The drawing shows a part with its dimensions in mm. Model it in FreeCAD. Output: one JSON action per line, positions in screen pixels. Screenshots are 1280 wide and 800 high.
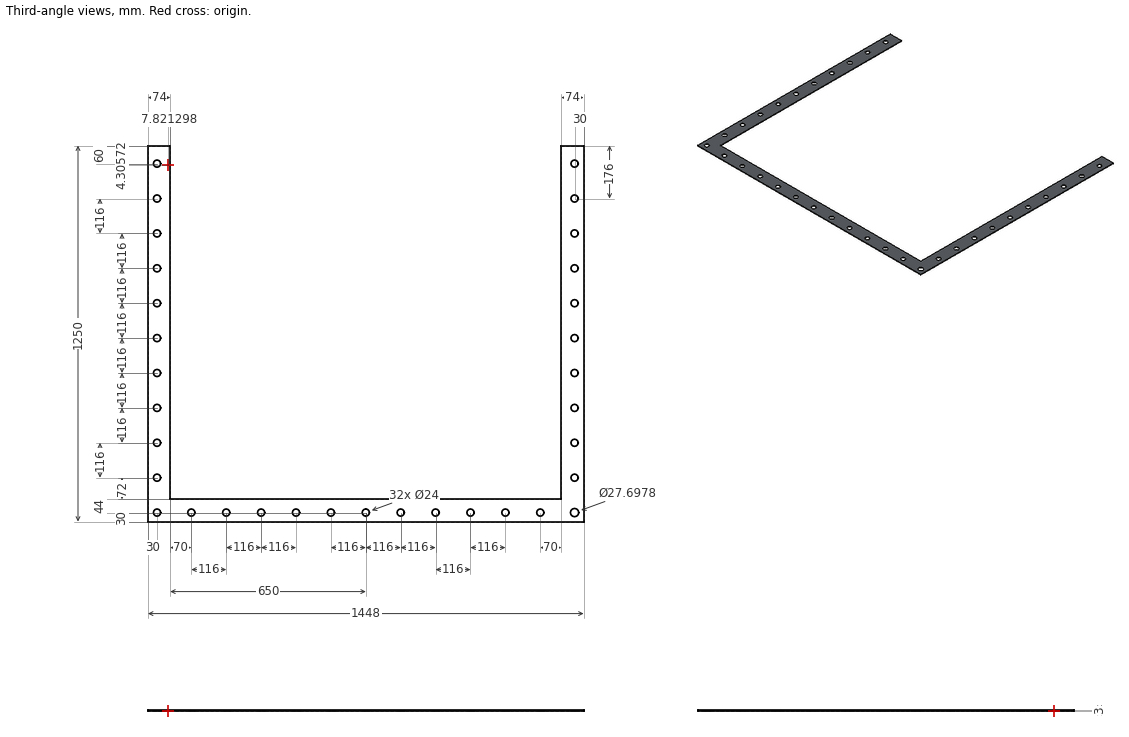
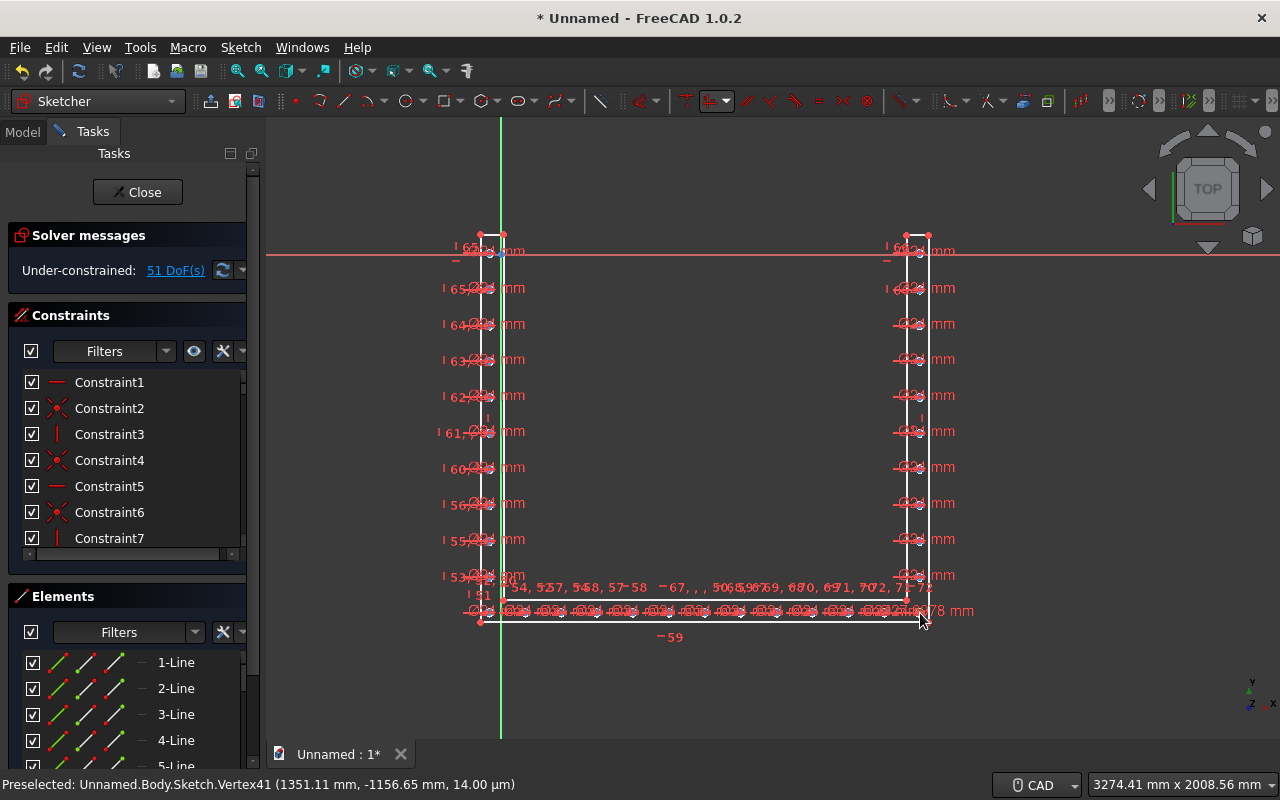
{"action": "left_click", "coordinate": [920, 577]}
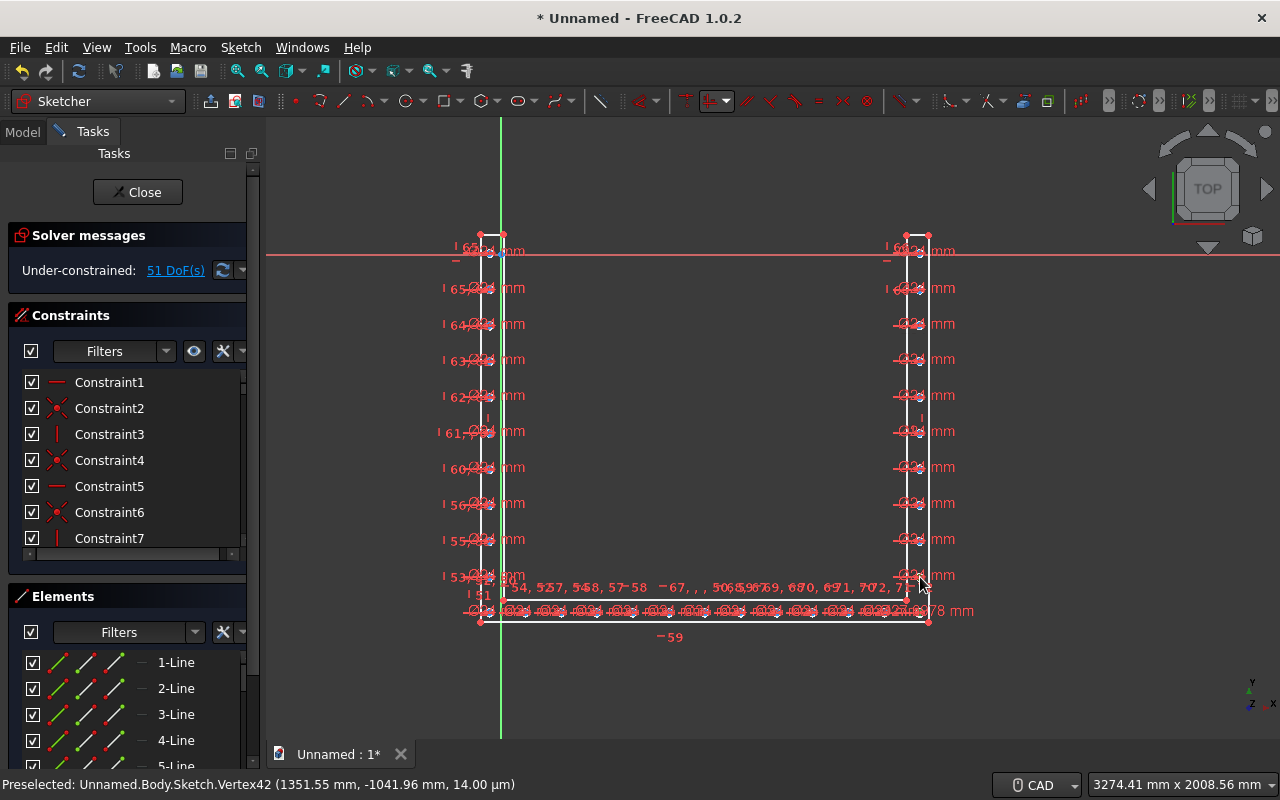
{"action": "left_click", "coordinate": [728, 102]}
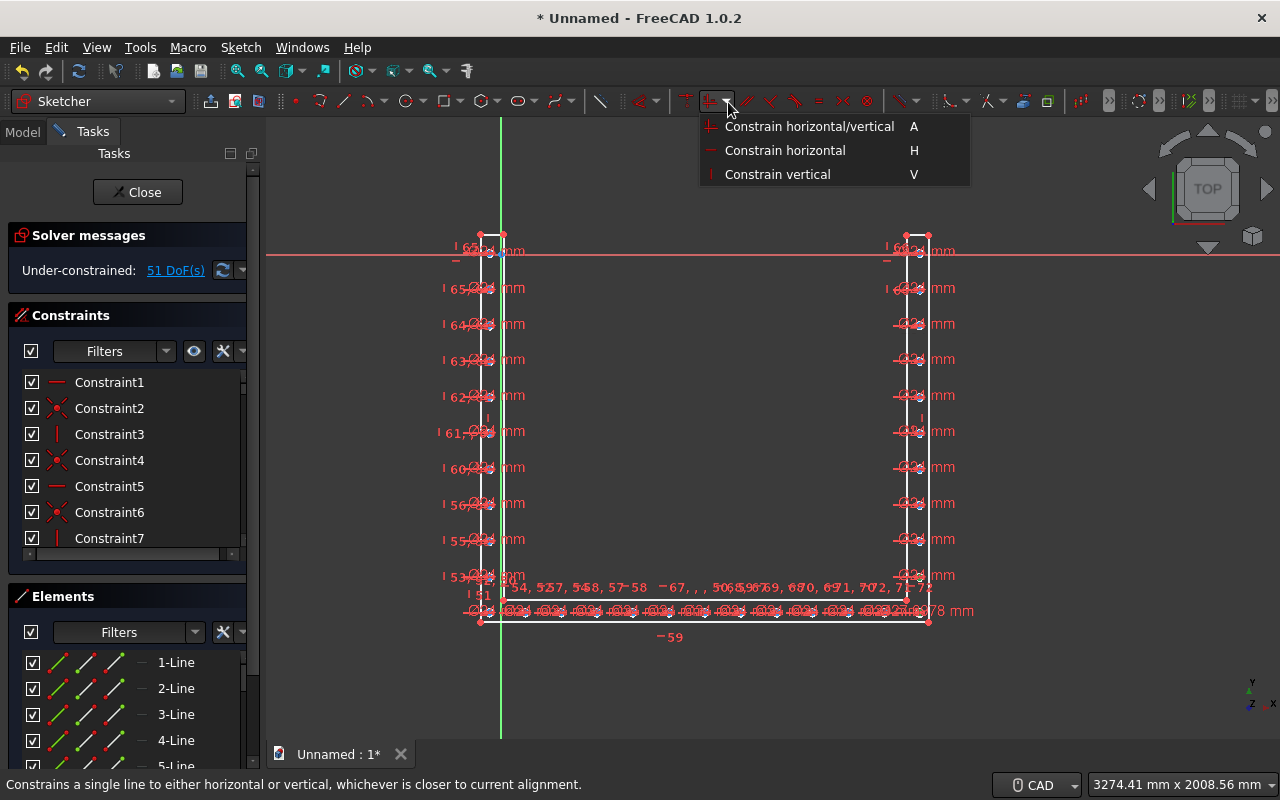
{"action": "left_click", "coordinate": [835, 174]}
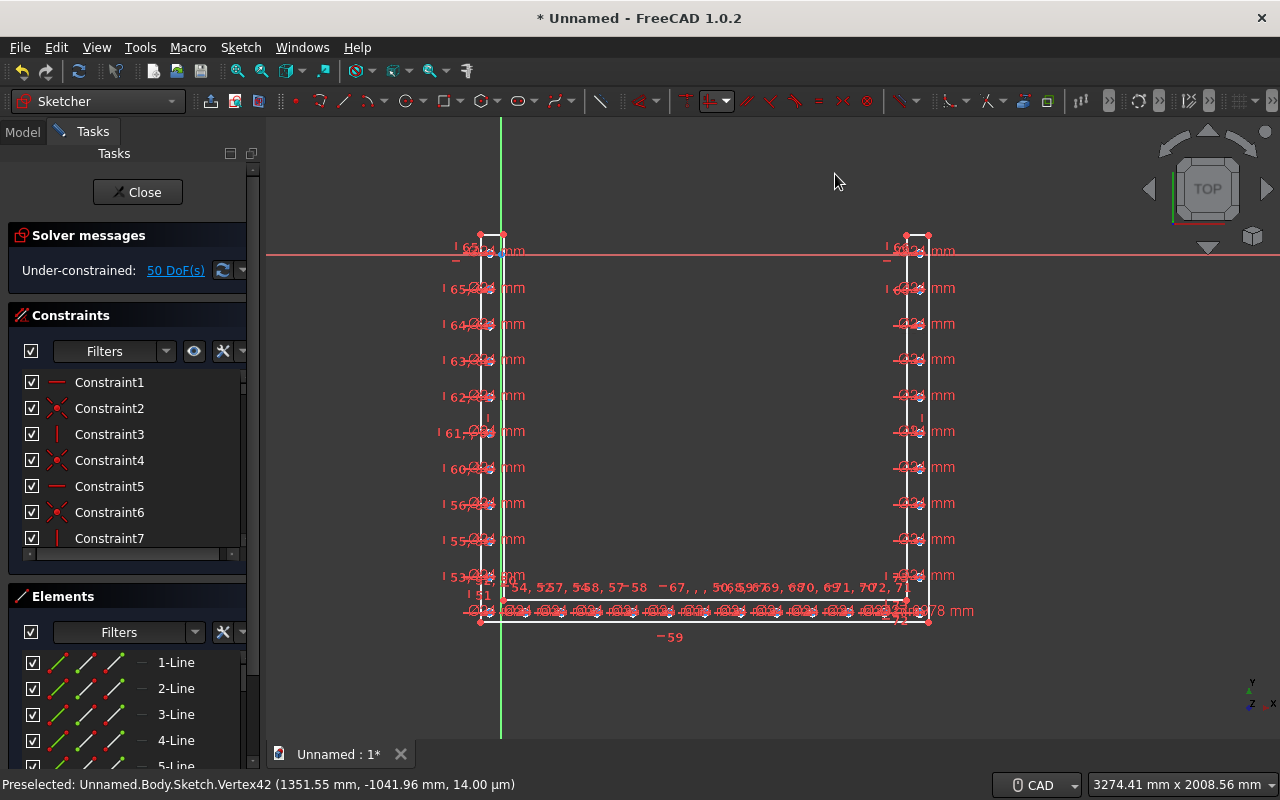
{"action": "left_click", "coordinate": [920, 577]}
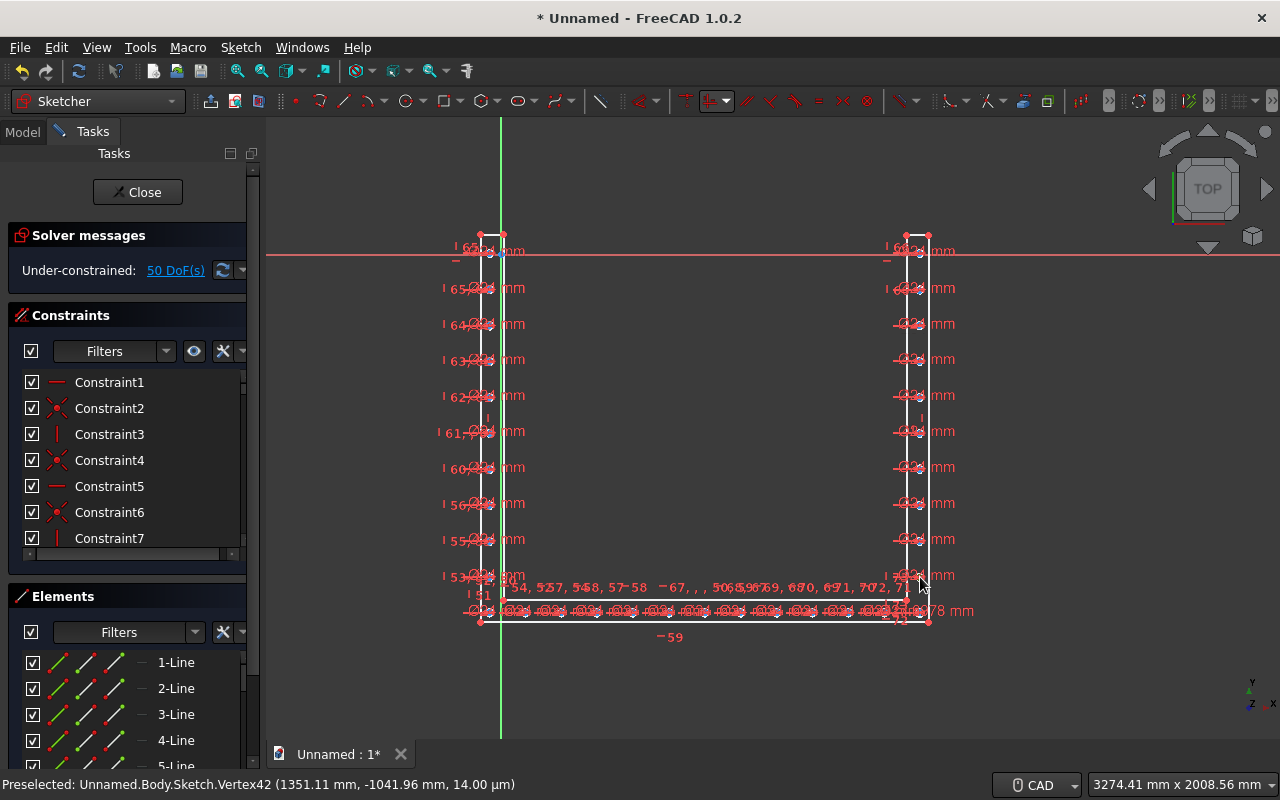
{"action": "left_click", "coordinate": [920, 541]}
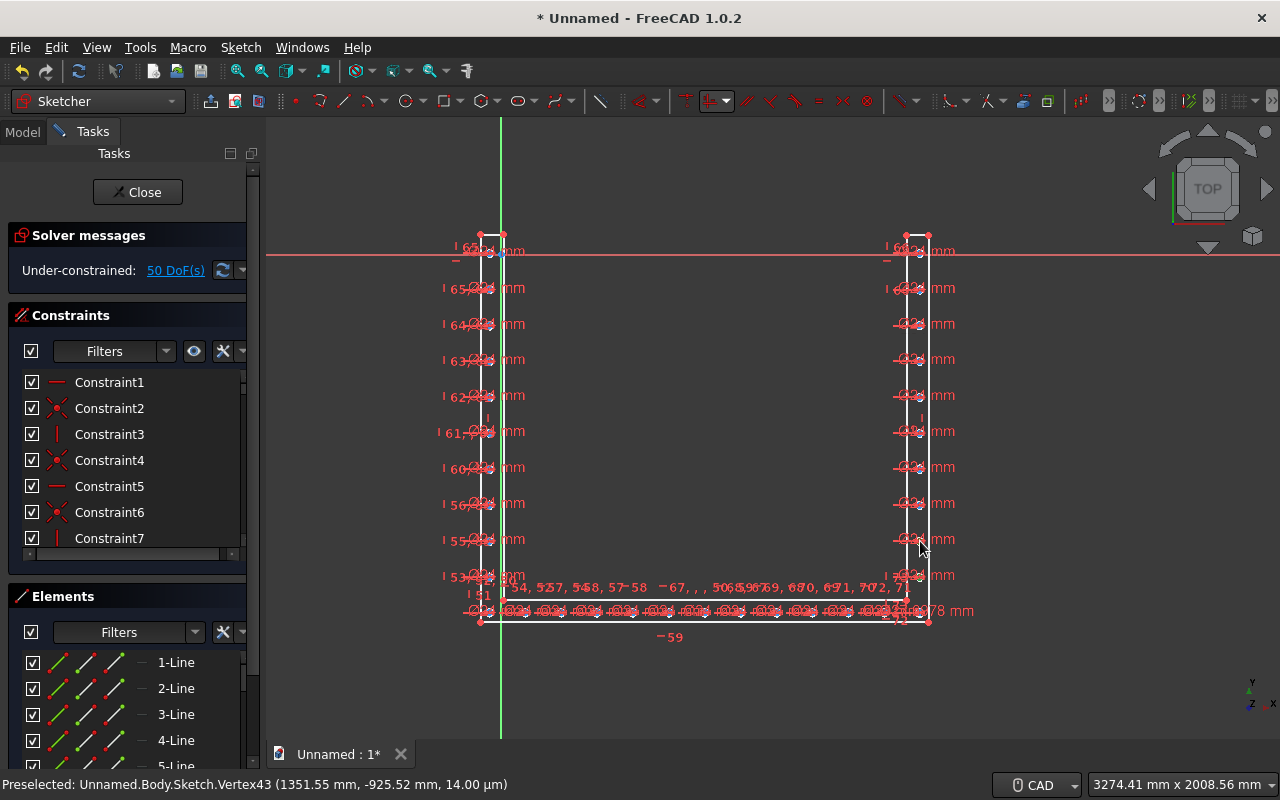
{"action": "left_click", "coordinate": [728, 102]}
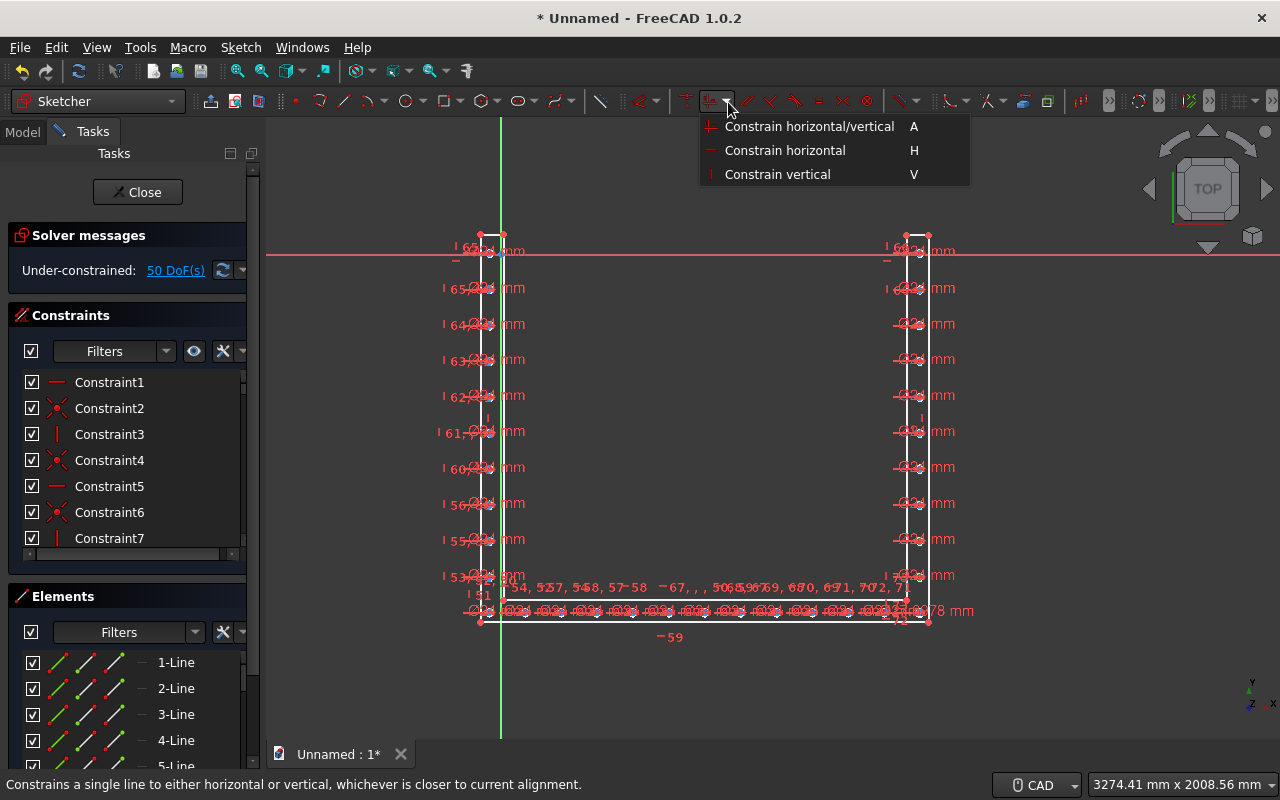
{"action": "left_click", "coordinate": [835, 174]}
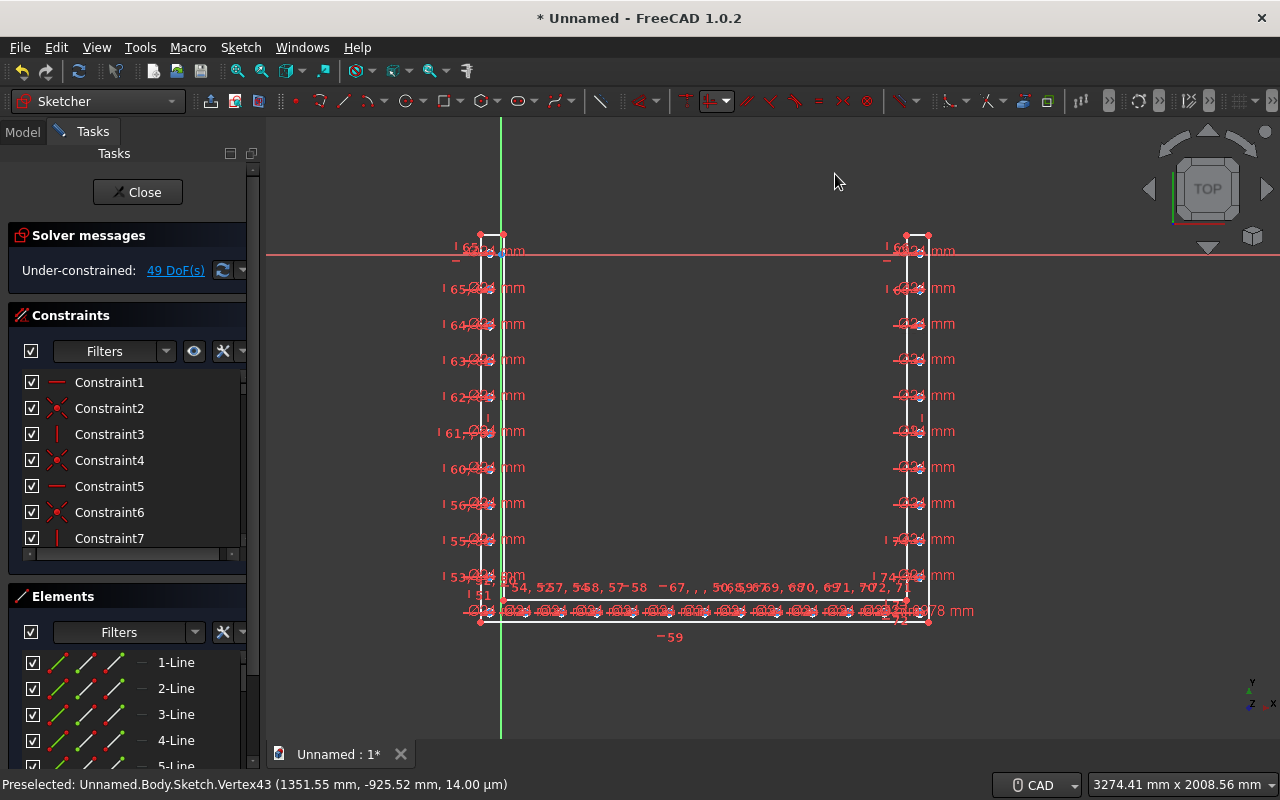
{"action": "left_click", "coordinate": [920, 541]}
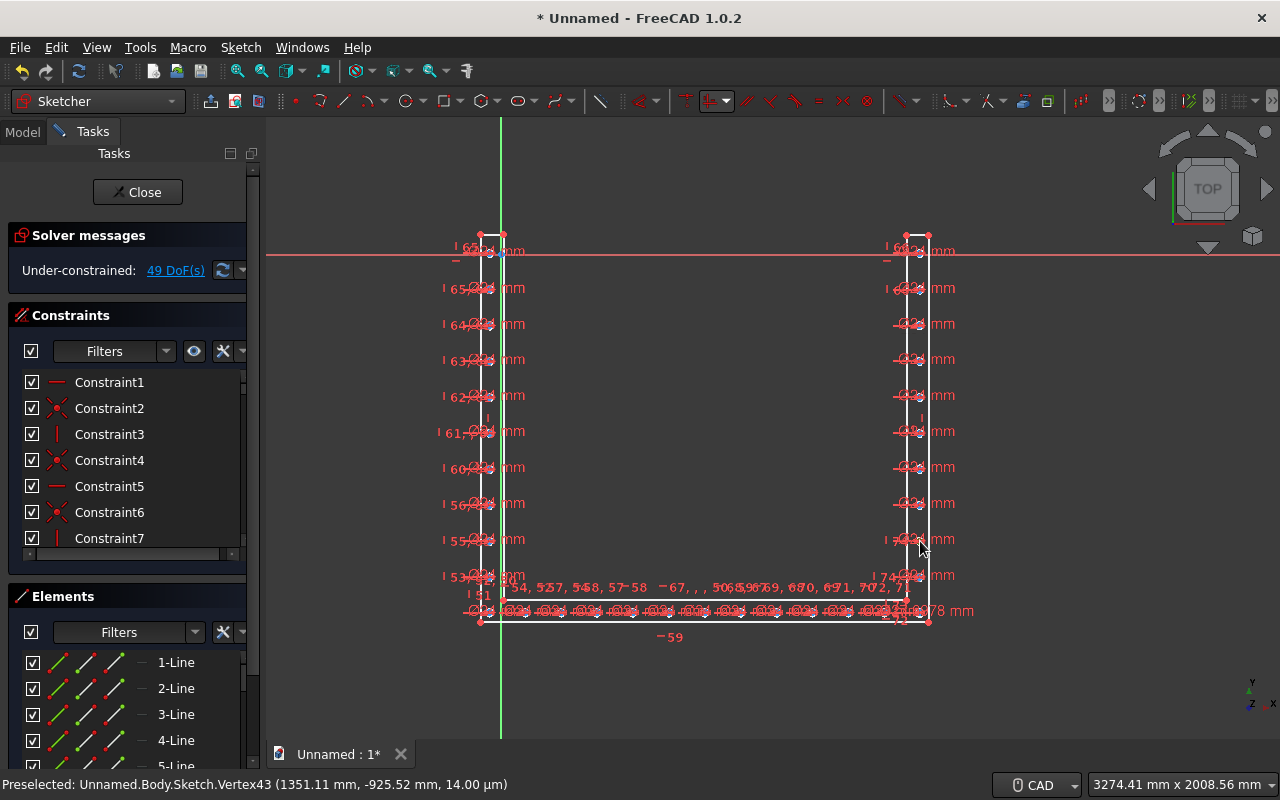
{"action": "left_click", "coordinate": [920, 505]}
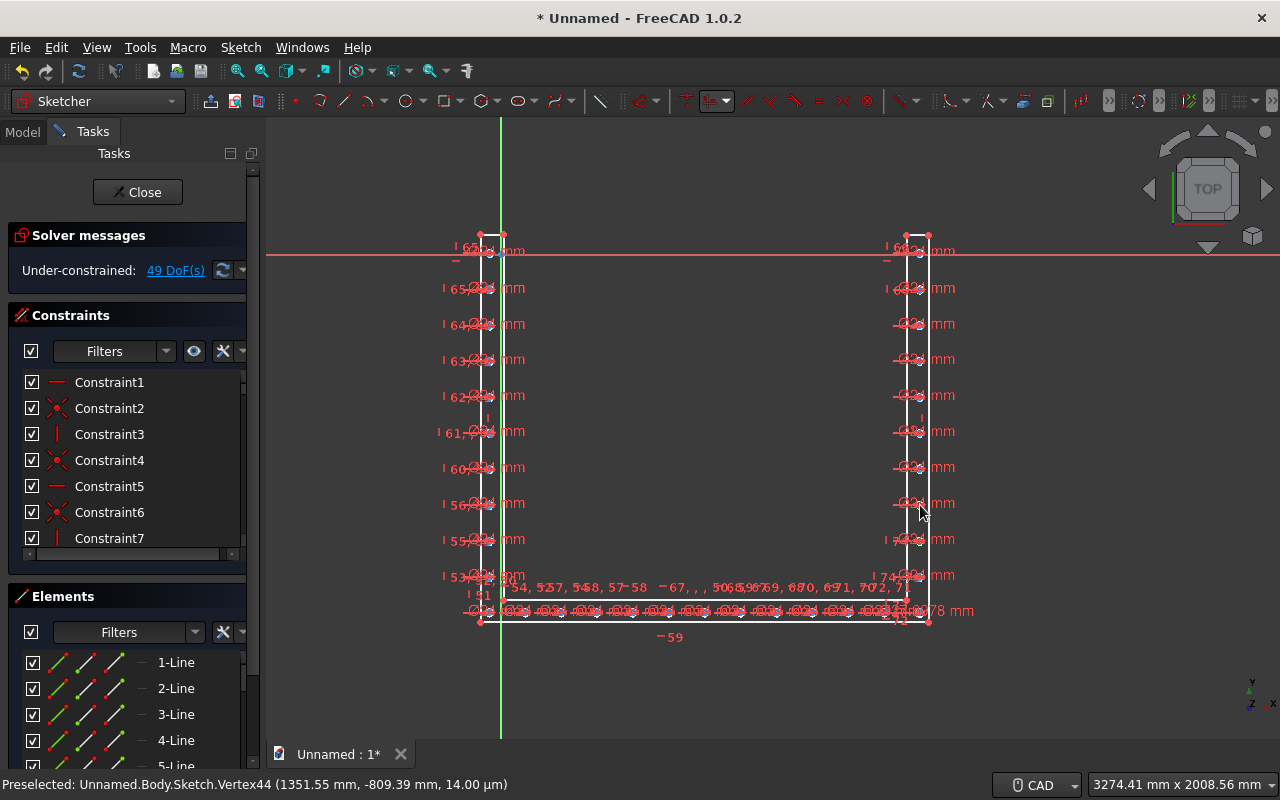
{"action": "left_click", "coordinate": [728, 102]}